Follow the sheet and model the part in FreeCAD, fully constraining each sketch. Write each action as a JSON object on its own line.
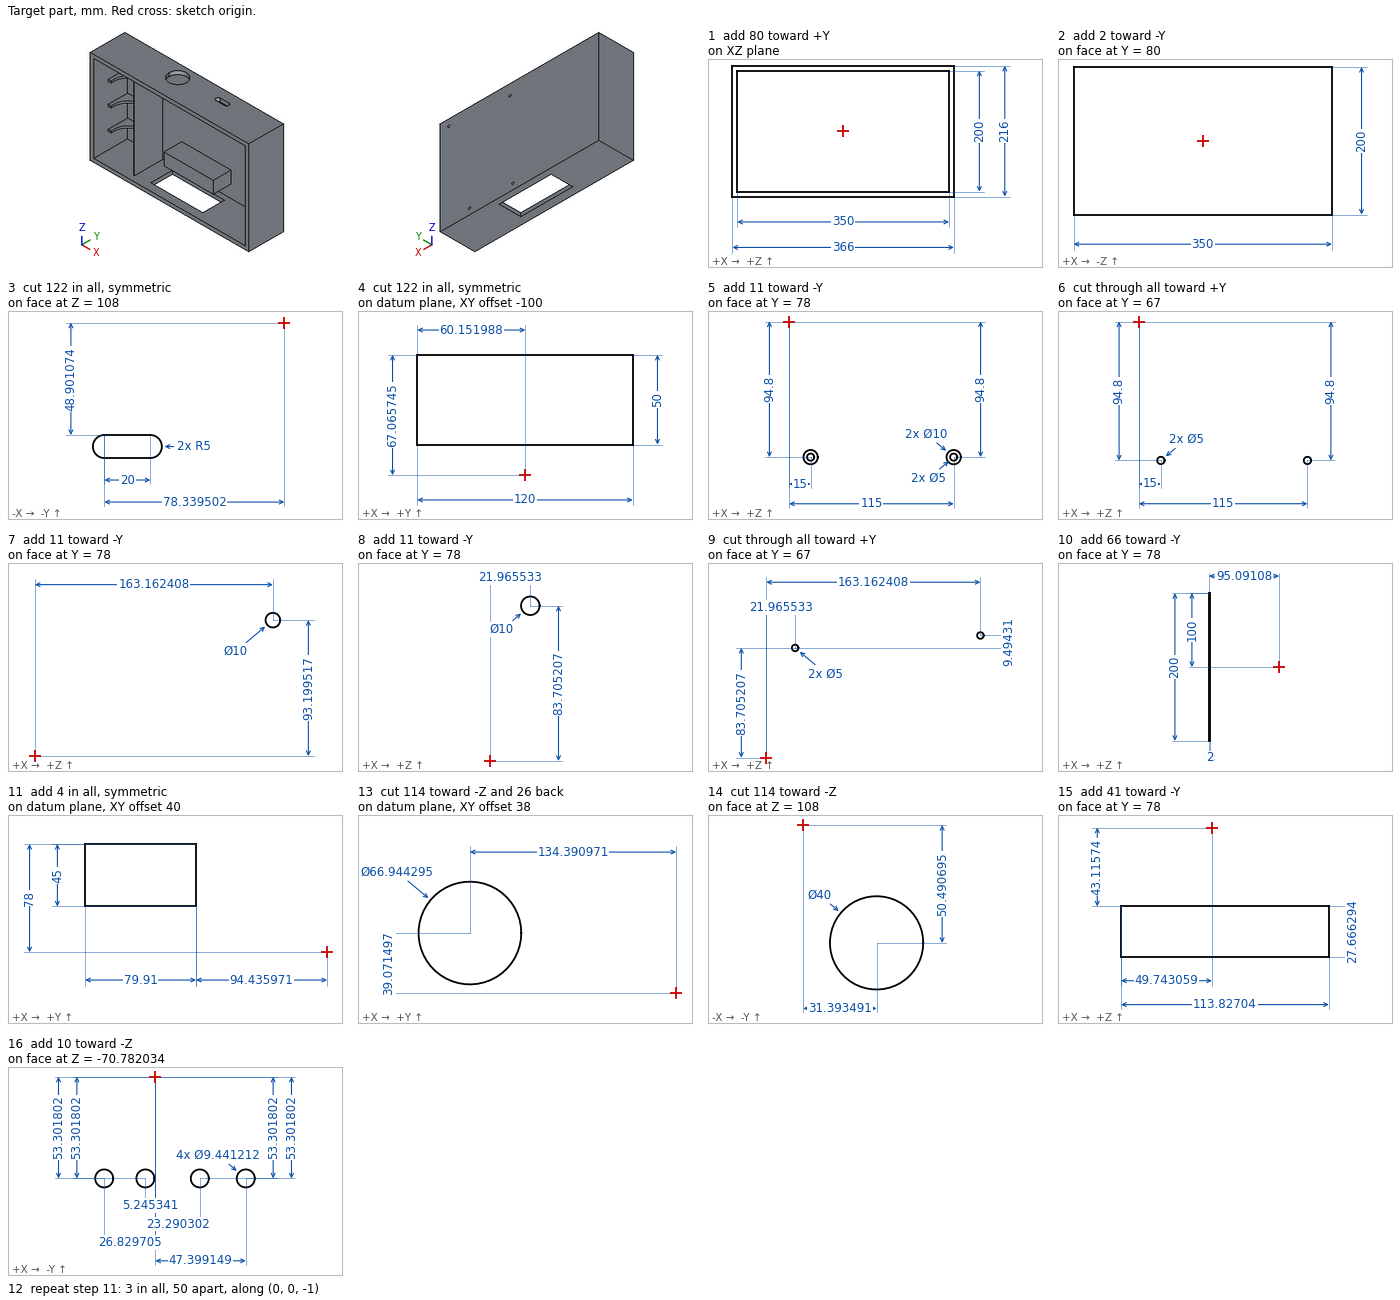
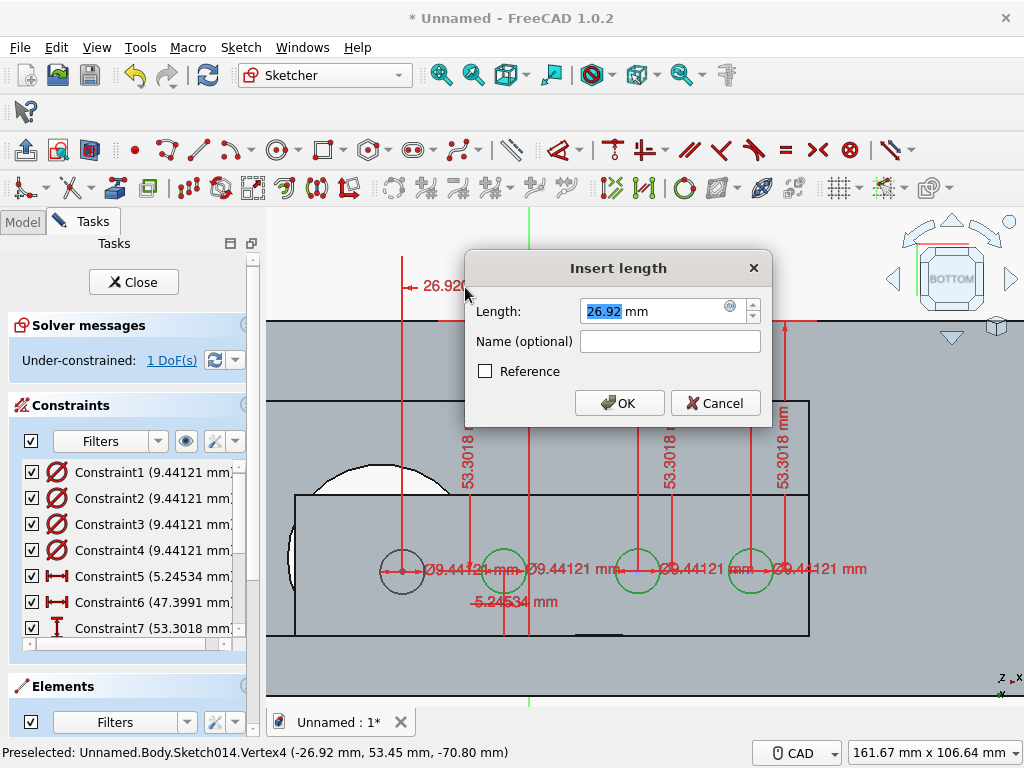
{"action": "type", "text": "26.829705"}
{"action": "key", "text": "Return"}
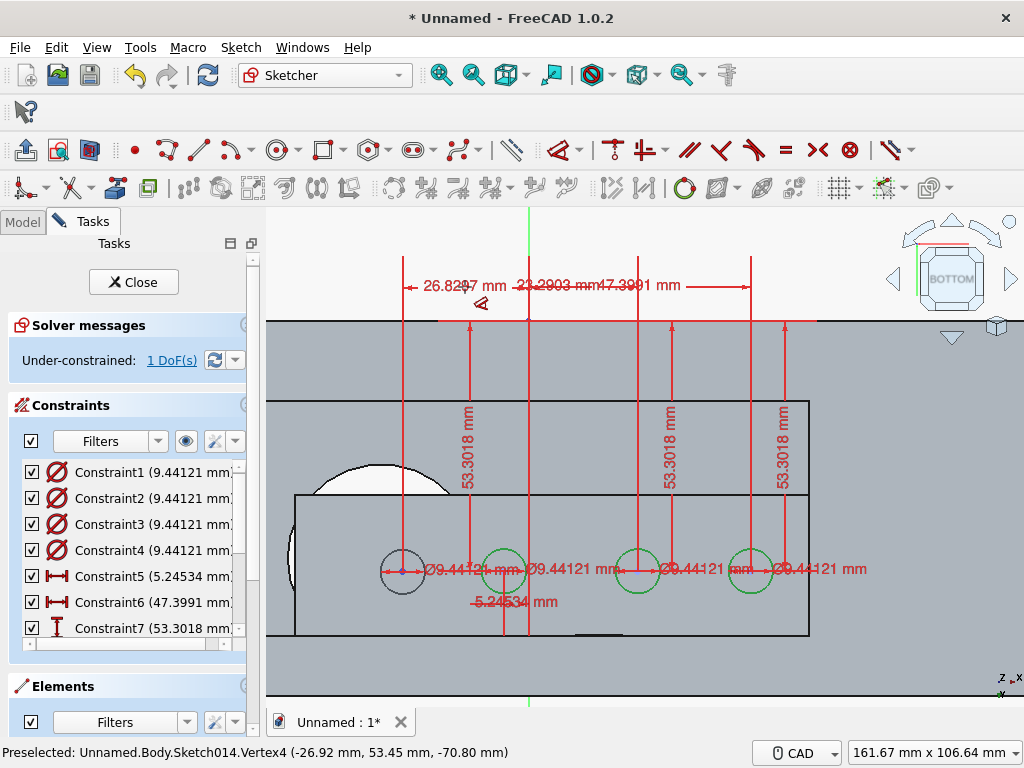
{"action": "left_click", "coordinate": [403, 572]}
{"action": "left_click", "coordinate": [369, 447]}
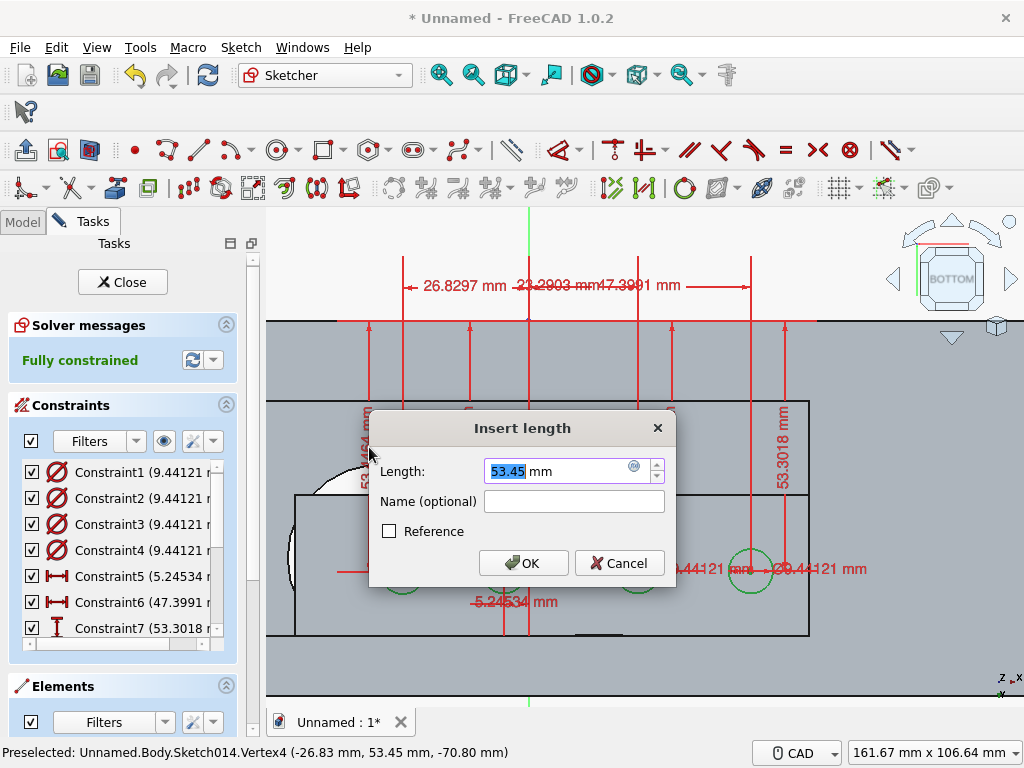
{"action": "type", "text": "53.301802"}
{"action": "key", "text": "Return"}
{"action": "key", "text": "Escape"}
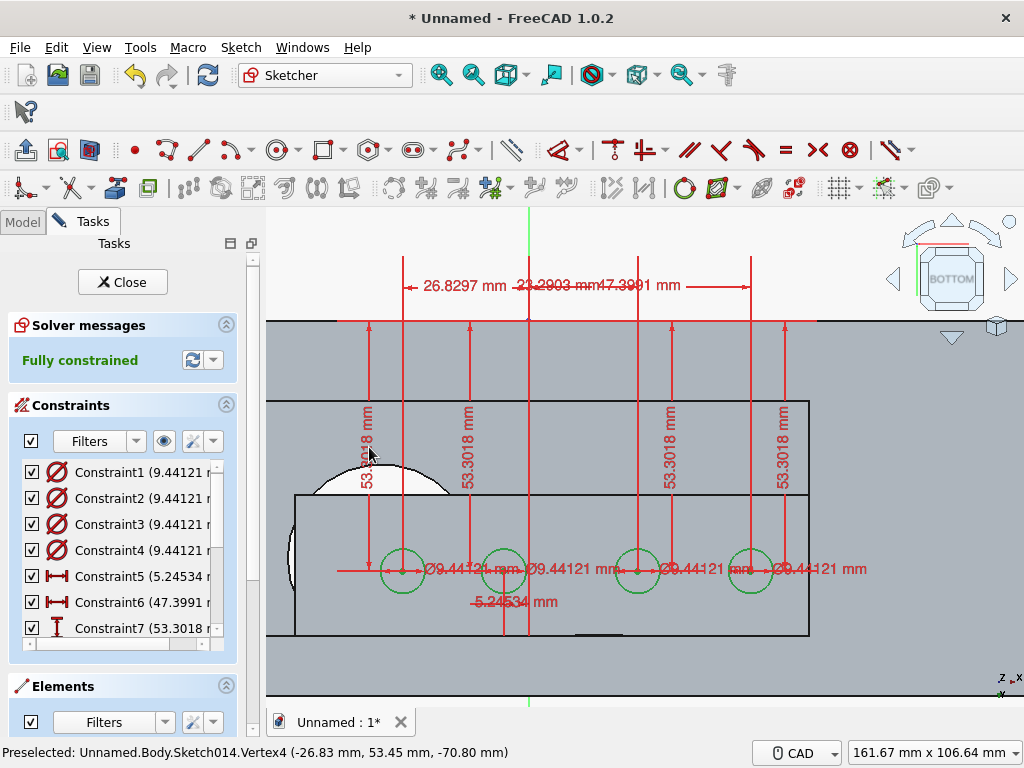
{"action": "left_click", "coordinate": [123, 282]}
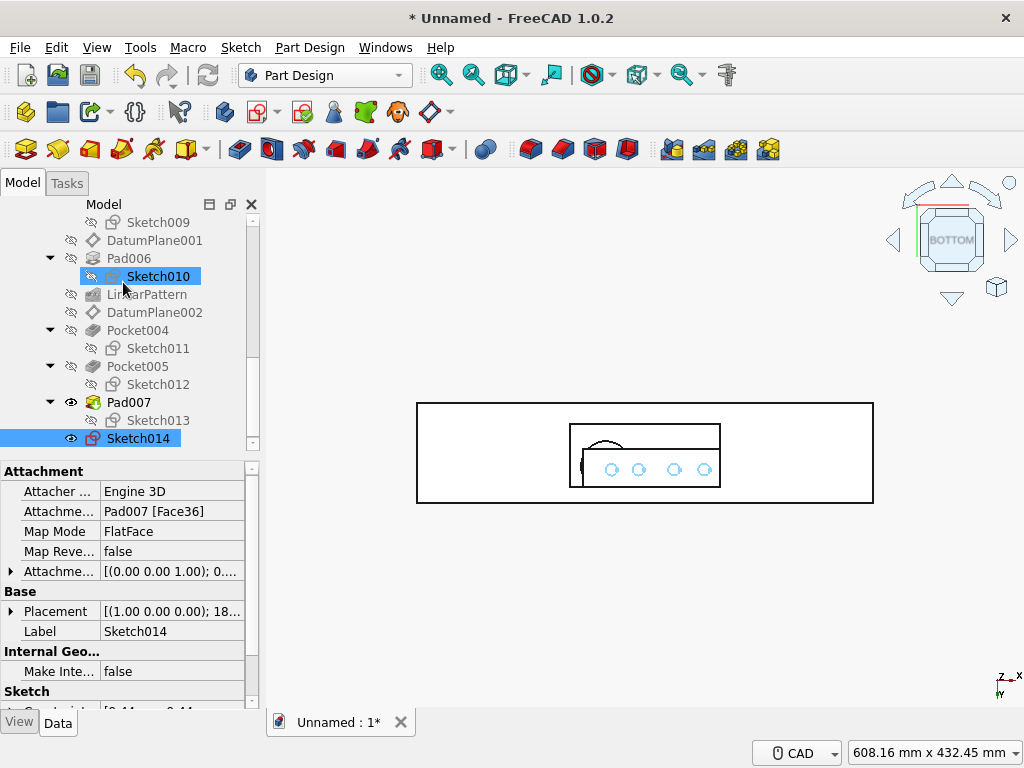
{"action": "left_click", "coordinate": [26, 150]}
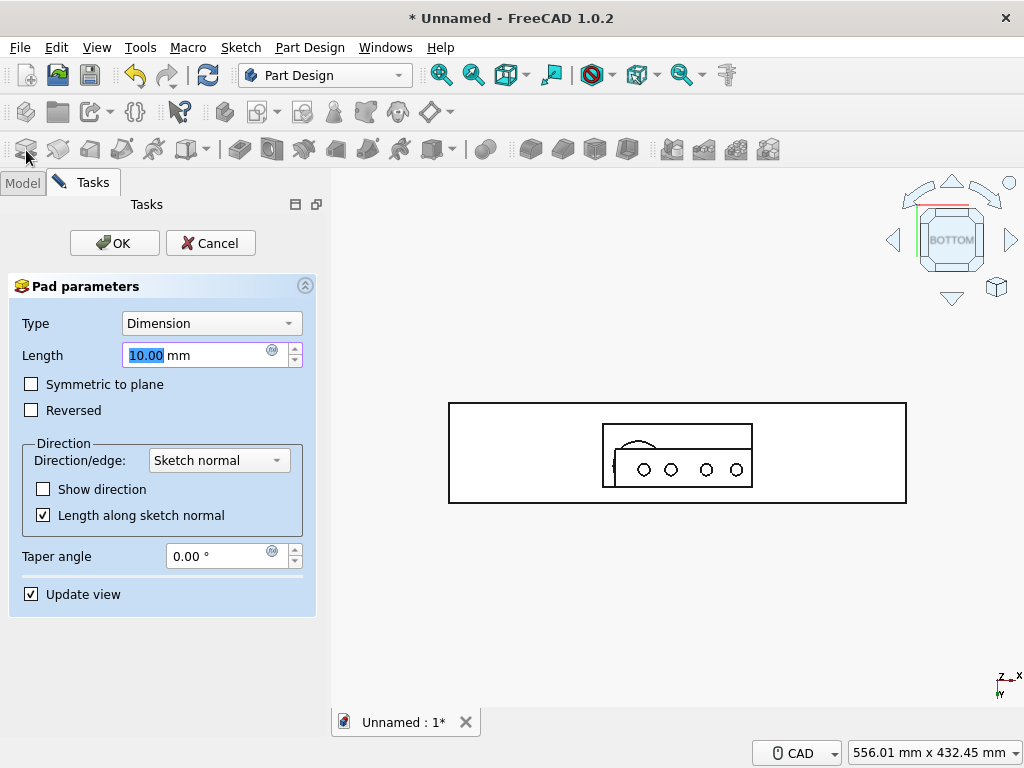
{"action": "type", "text": "10"}
{"action": "key", "text": "Tab"}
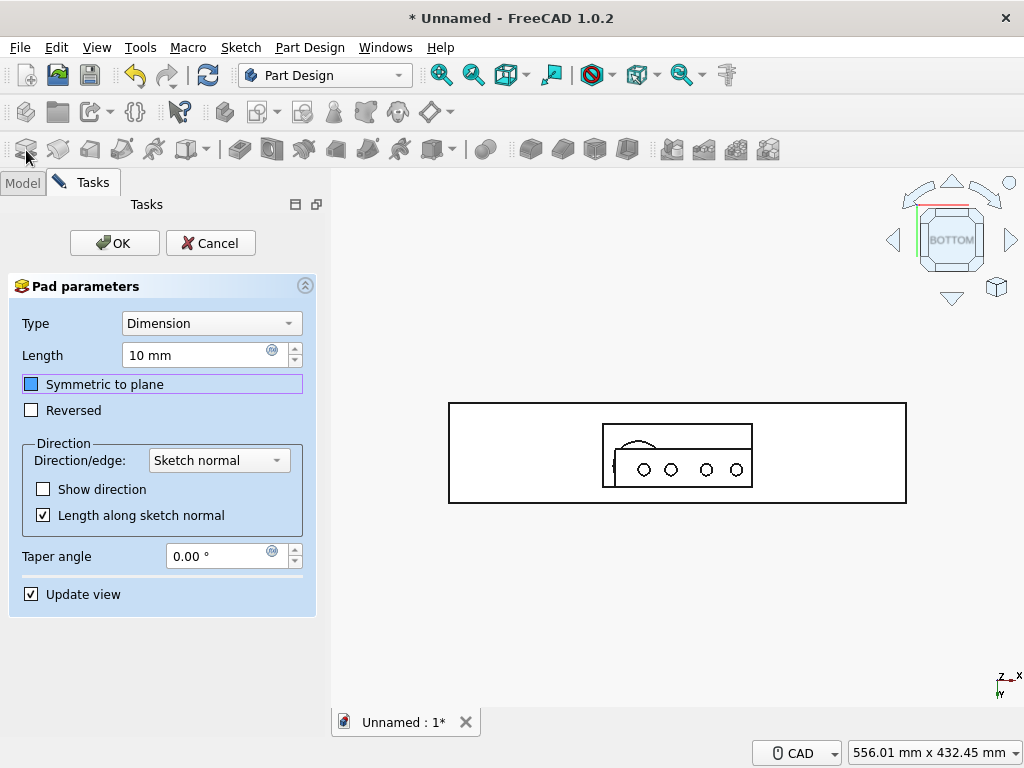
{"action": "left_click", "coordinate": [115, 243]}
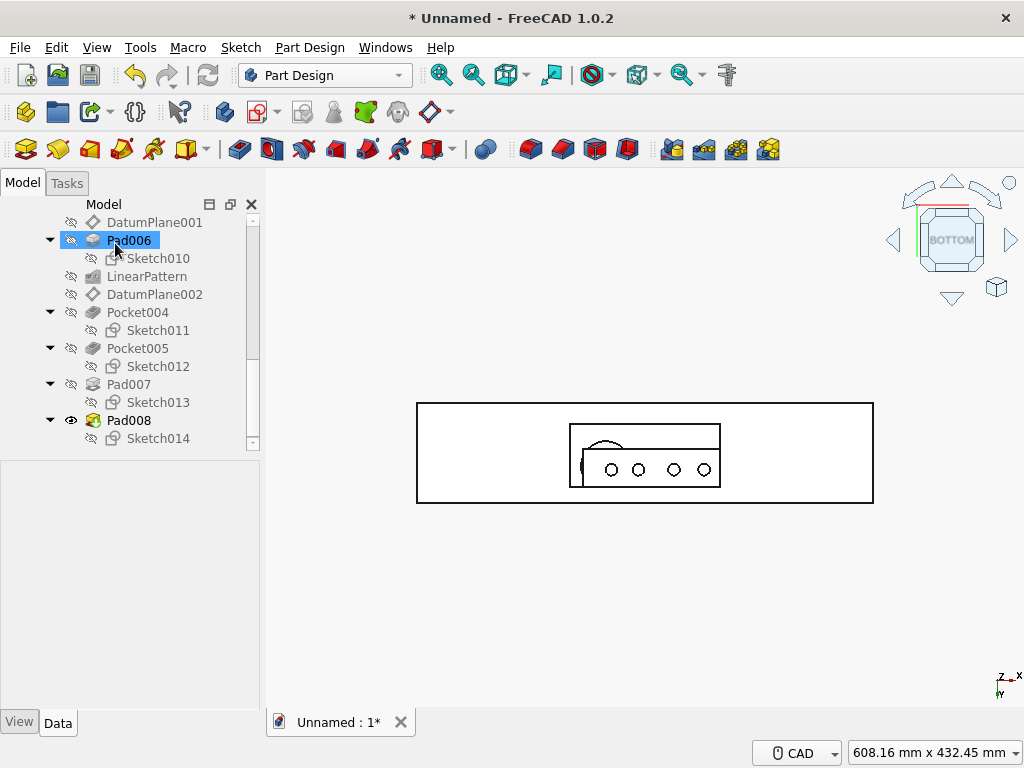
{"action": "key", "text": "0"}